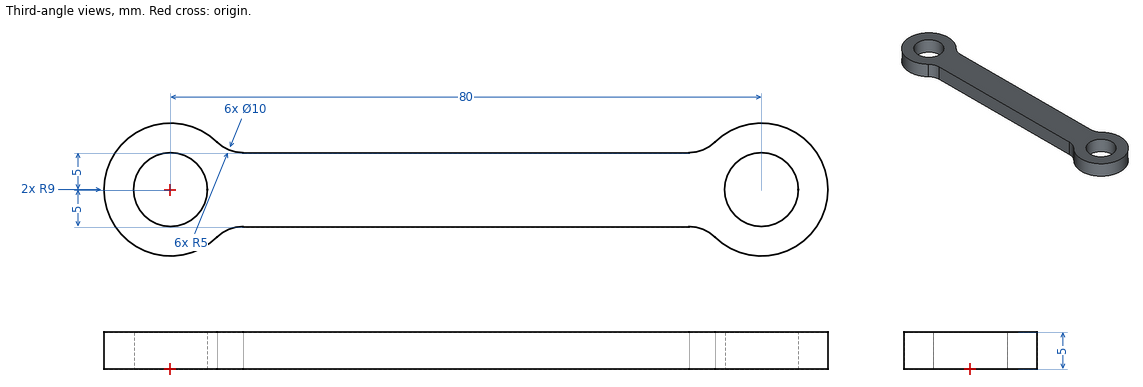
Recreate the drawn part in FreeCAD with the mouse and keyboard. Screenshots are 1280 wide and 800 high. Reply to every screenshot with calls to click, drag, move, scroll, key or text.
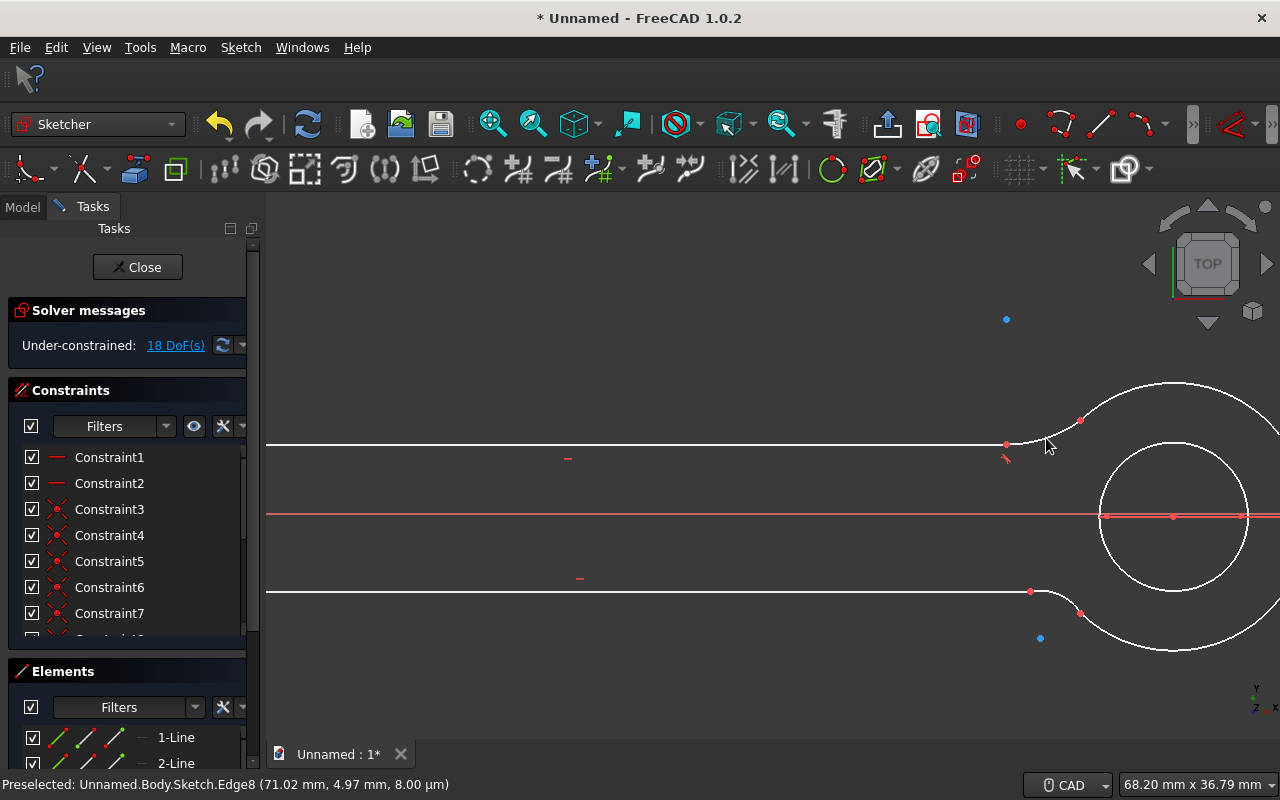
click(401, 592)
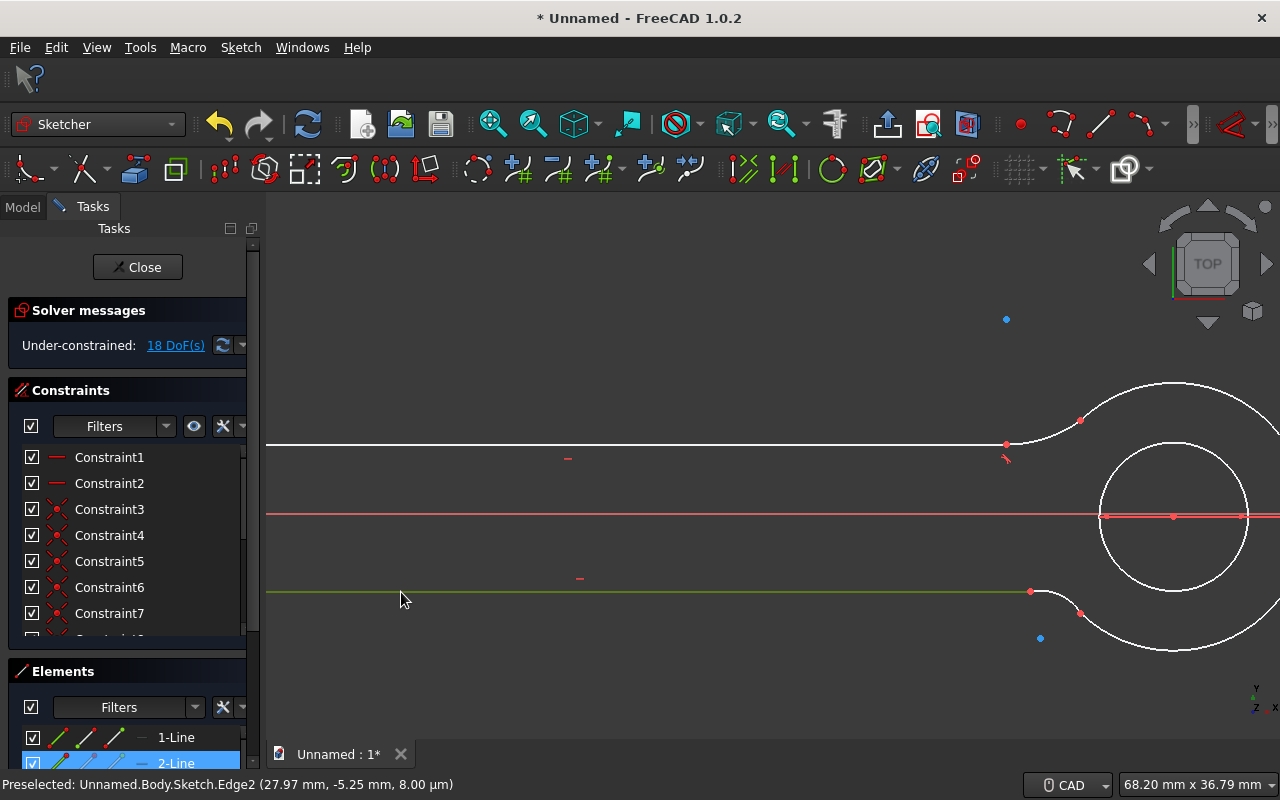
scroll(777, 437, down, 5)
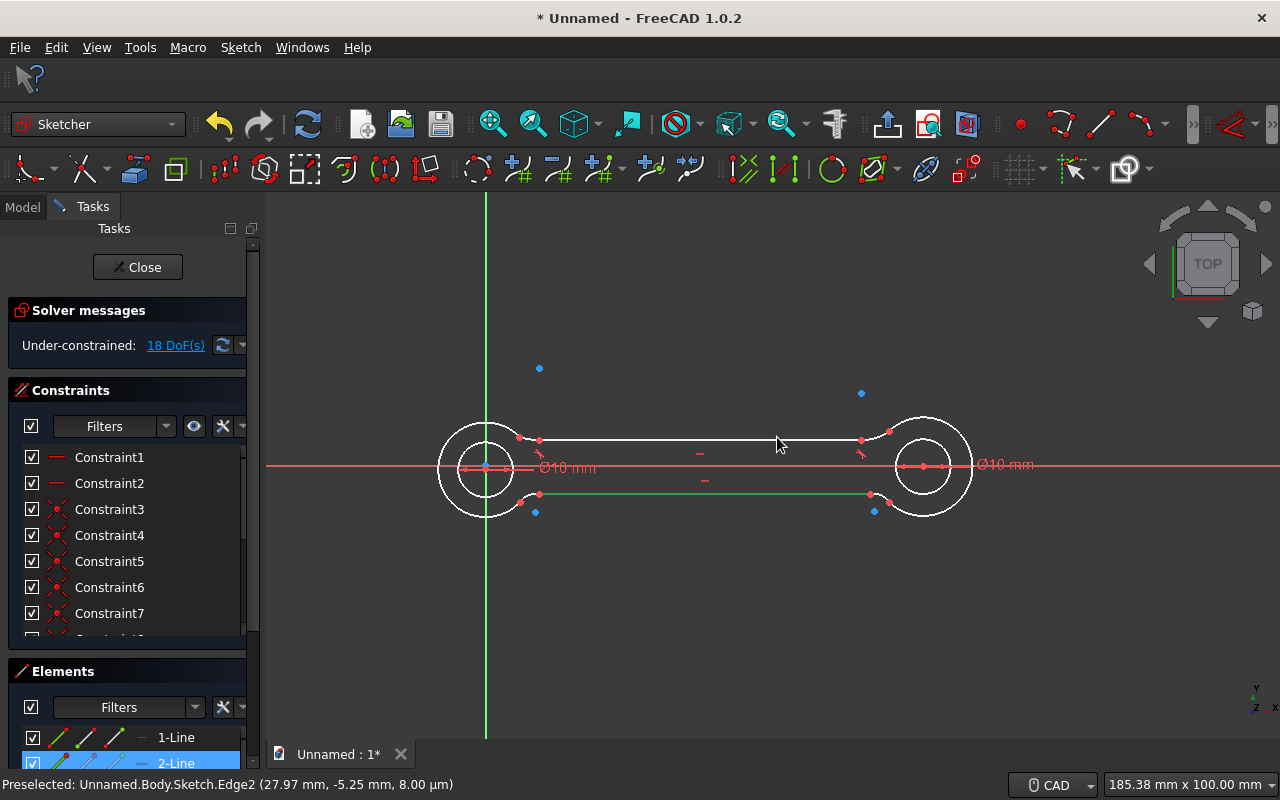
scroll(533, 494, up, 4)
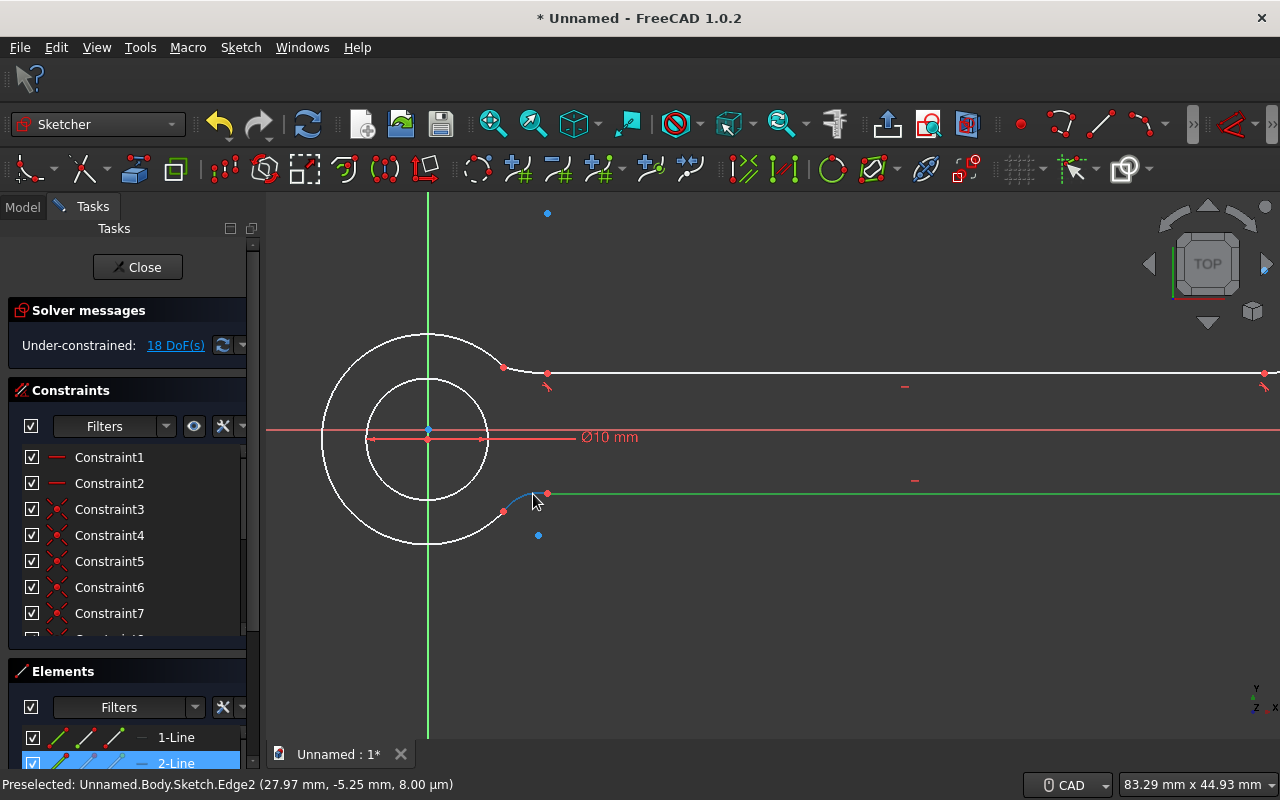
click(532, 493)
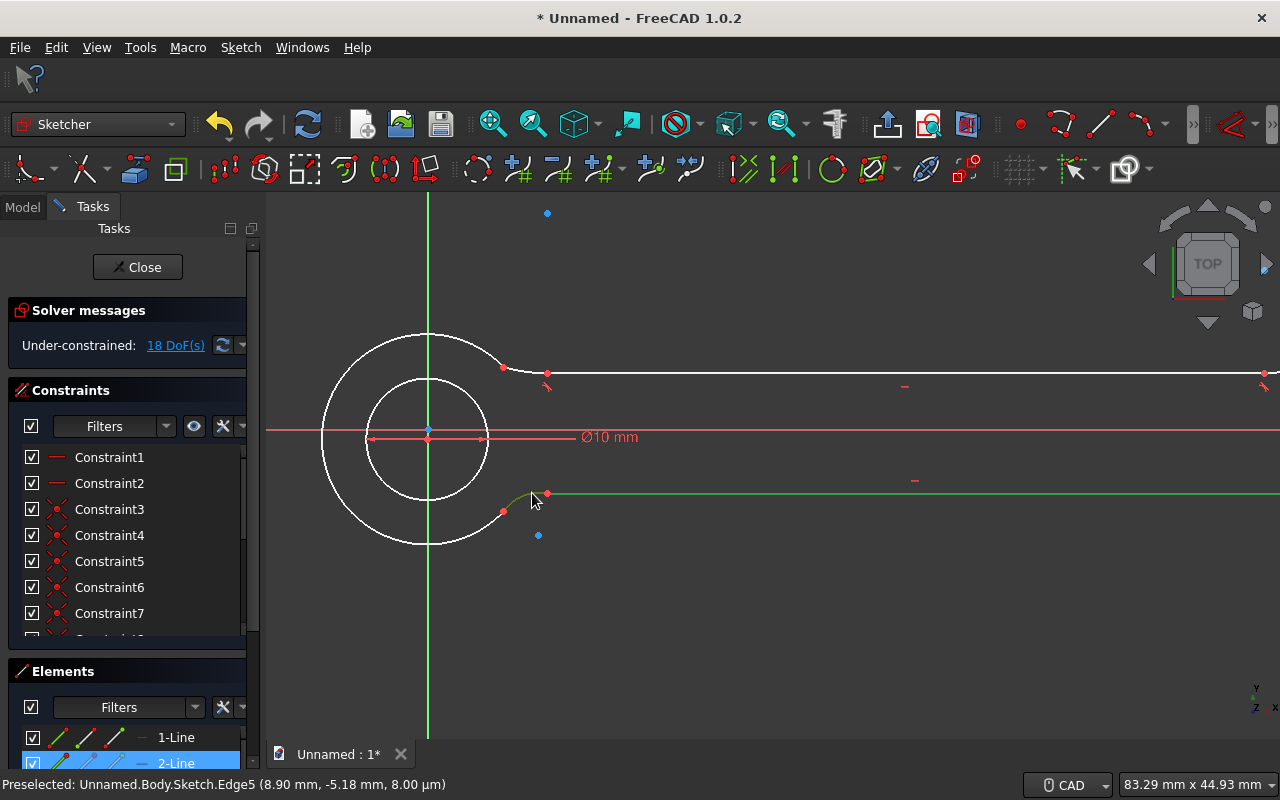
key(t)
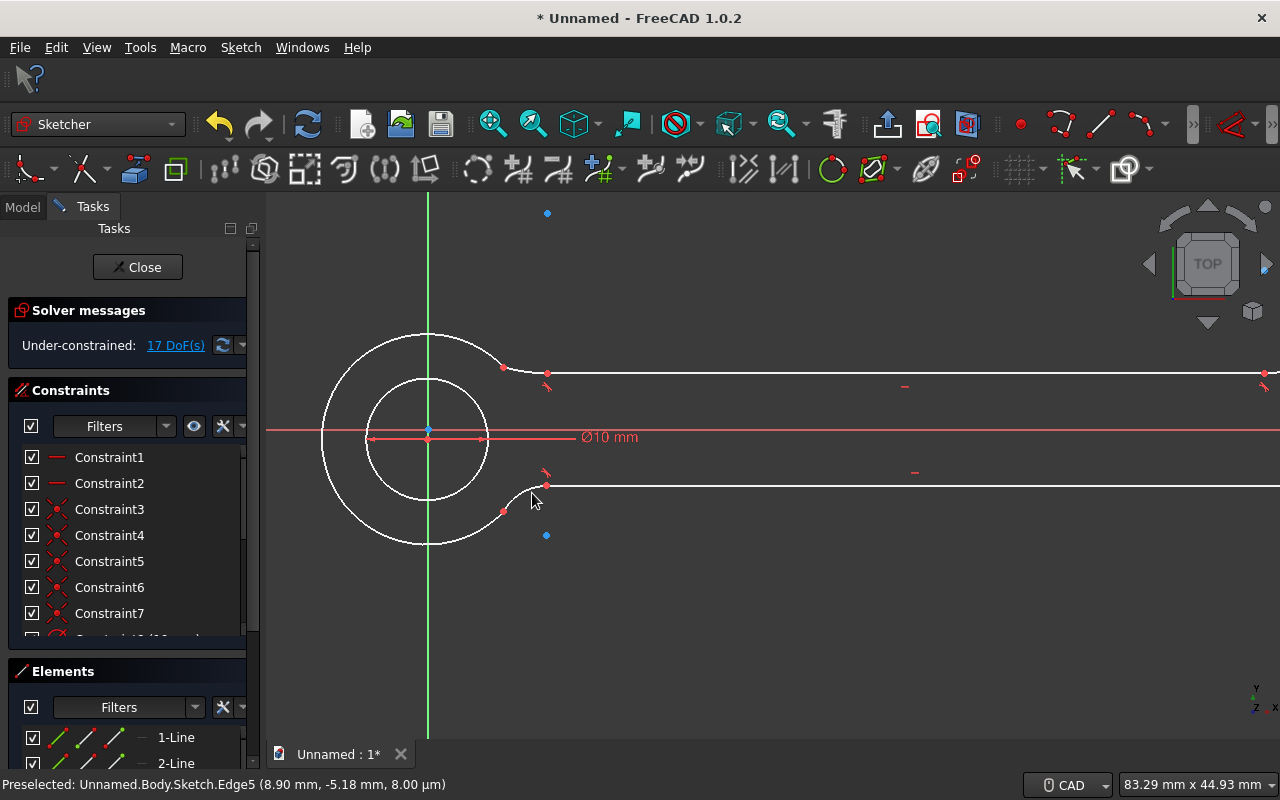
click(768, 486)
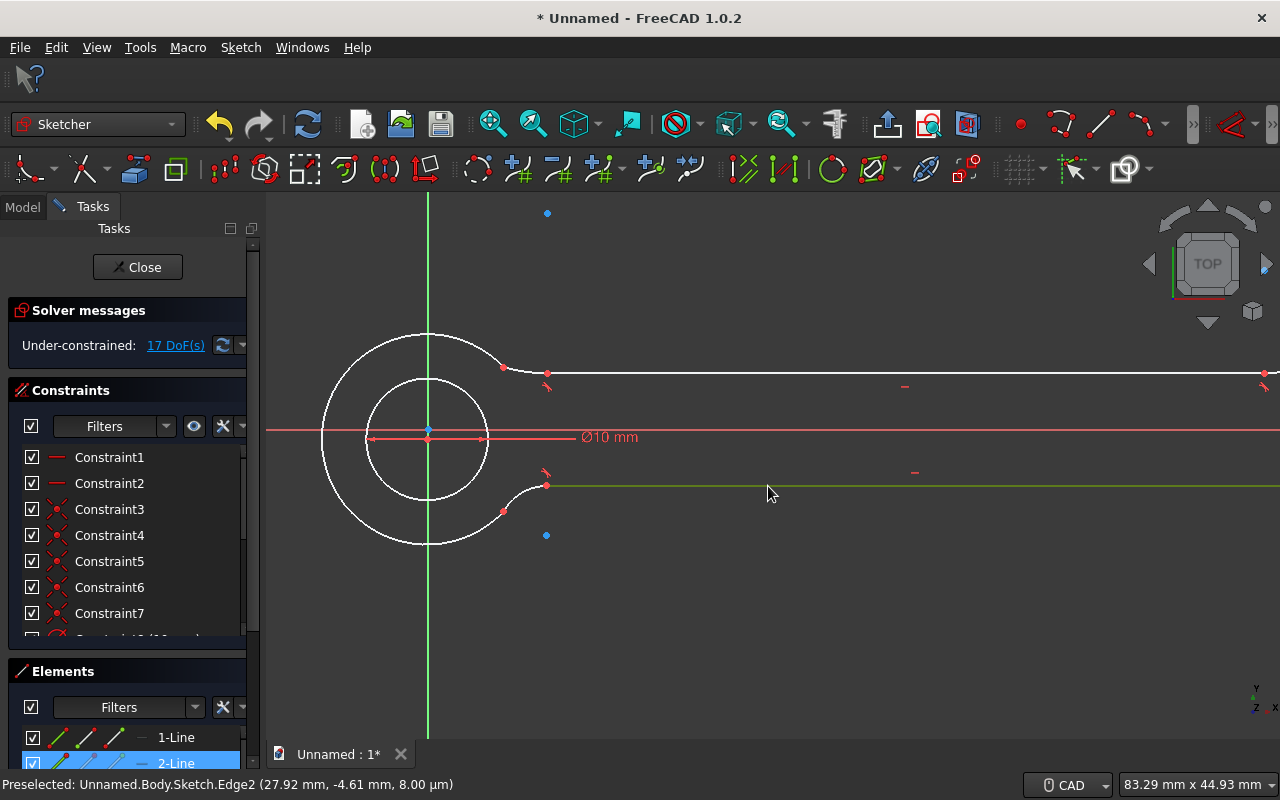
scroll(533, 495, down, 4)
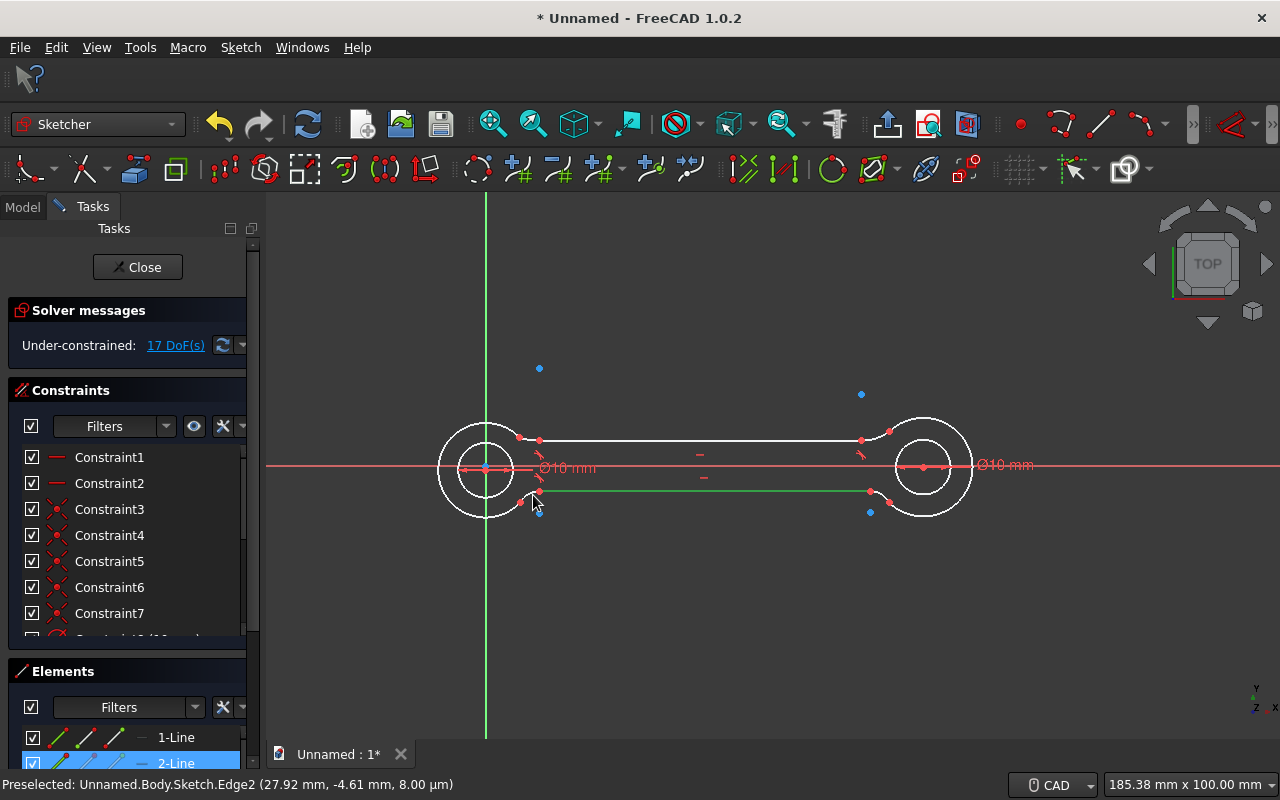
scroll(885, 497, up, 4)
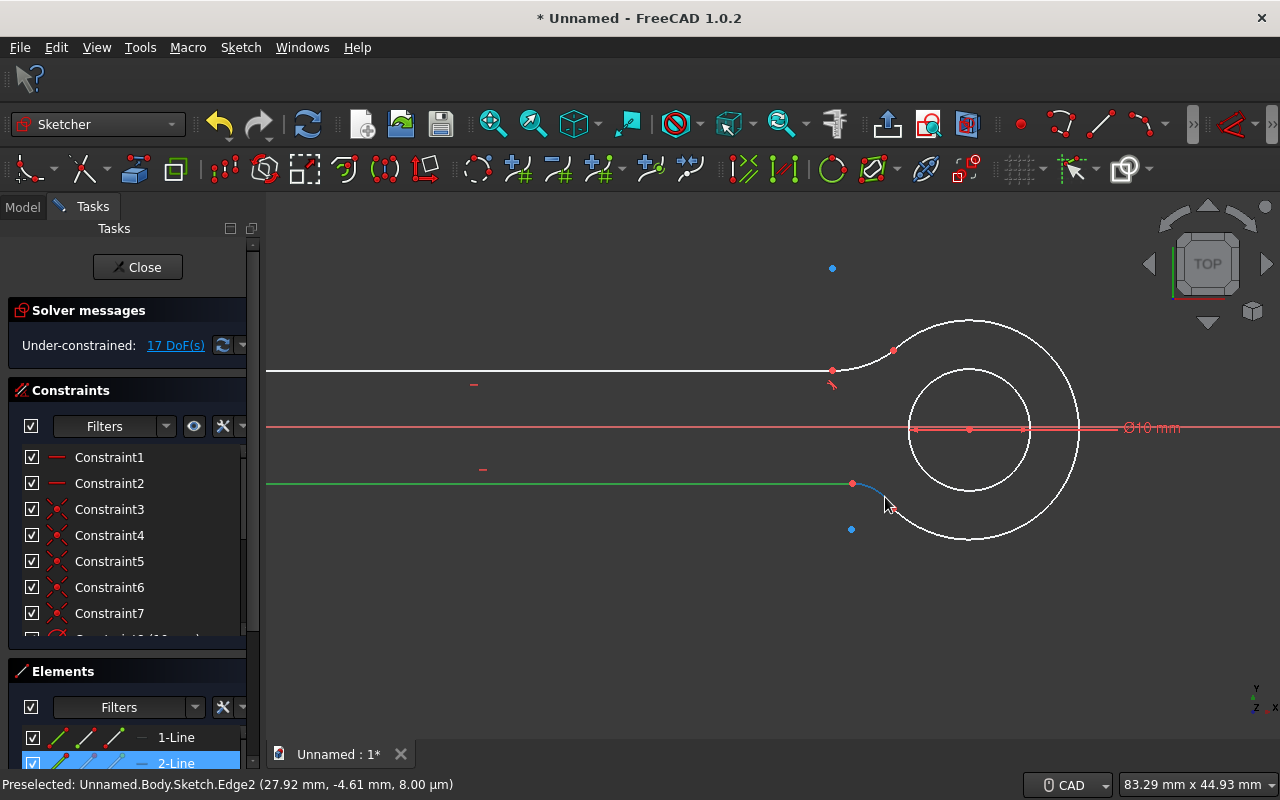
click(884, 497)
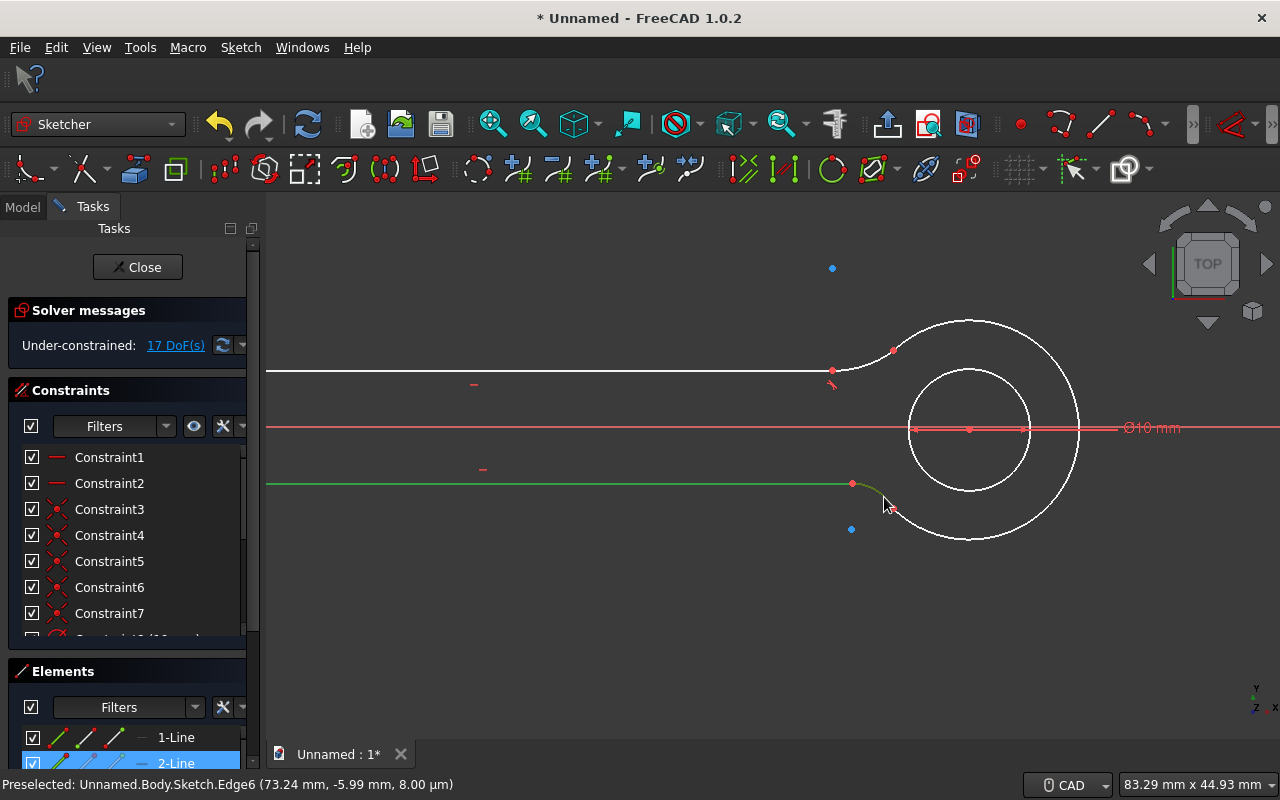
key(t)